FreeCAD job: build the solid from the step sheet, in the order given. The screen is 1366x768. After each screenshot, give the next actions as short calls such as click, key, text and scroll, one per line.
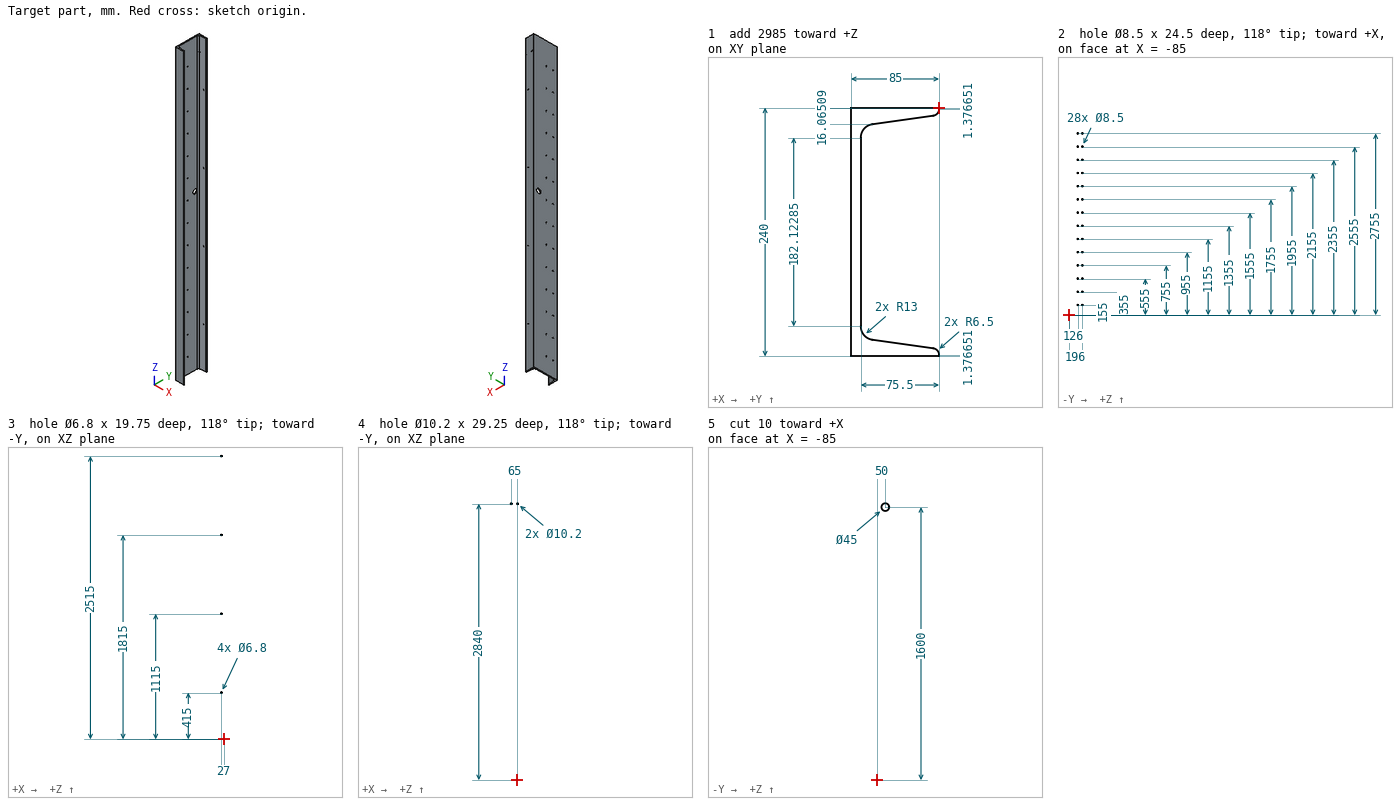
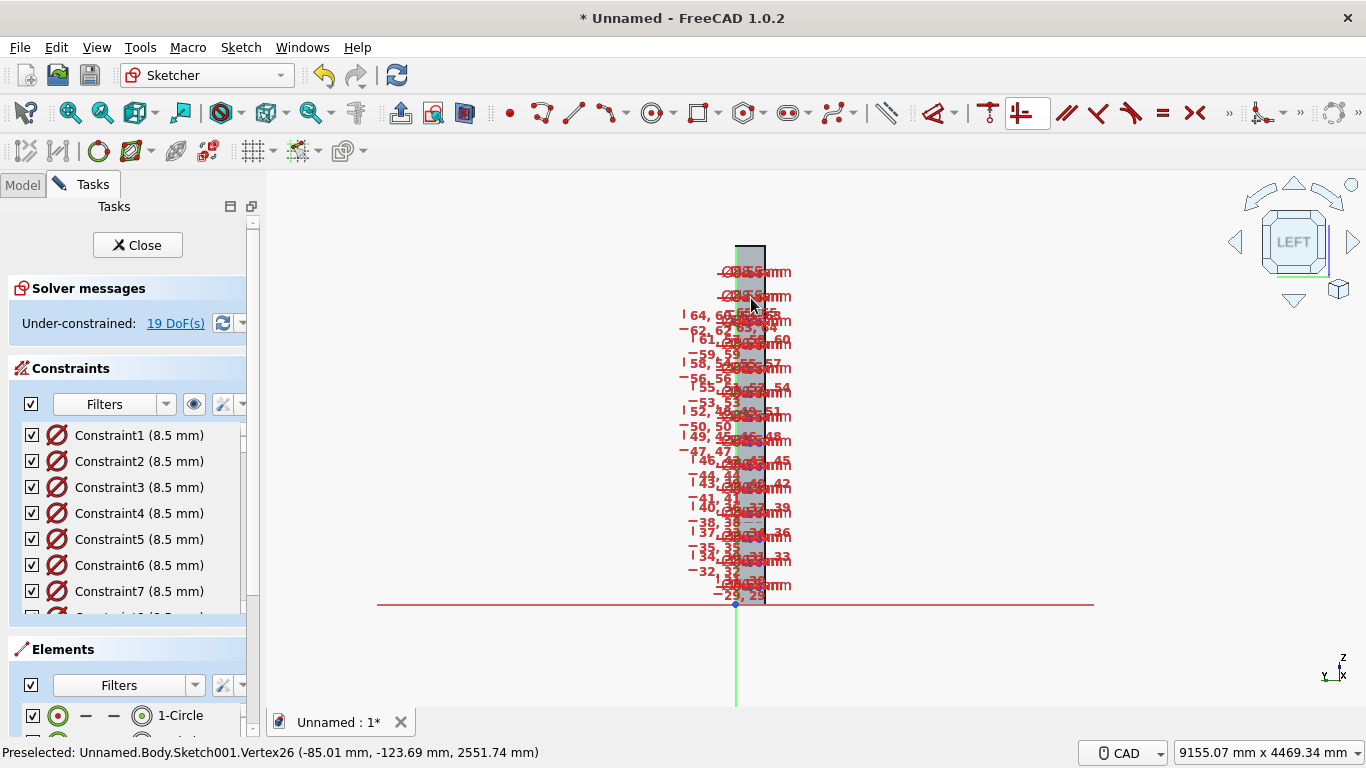
scroll(751, 298, up, 2)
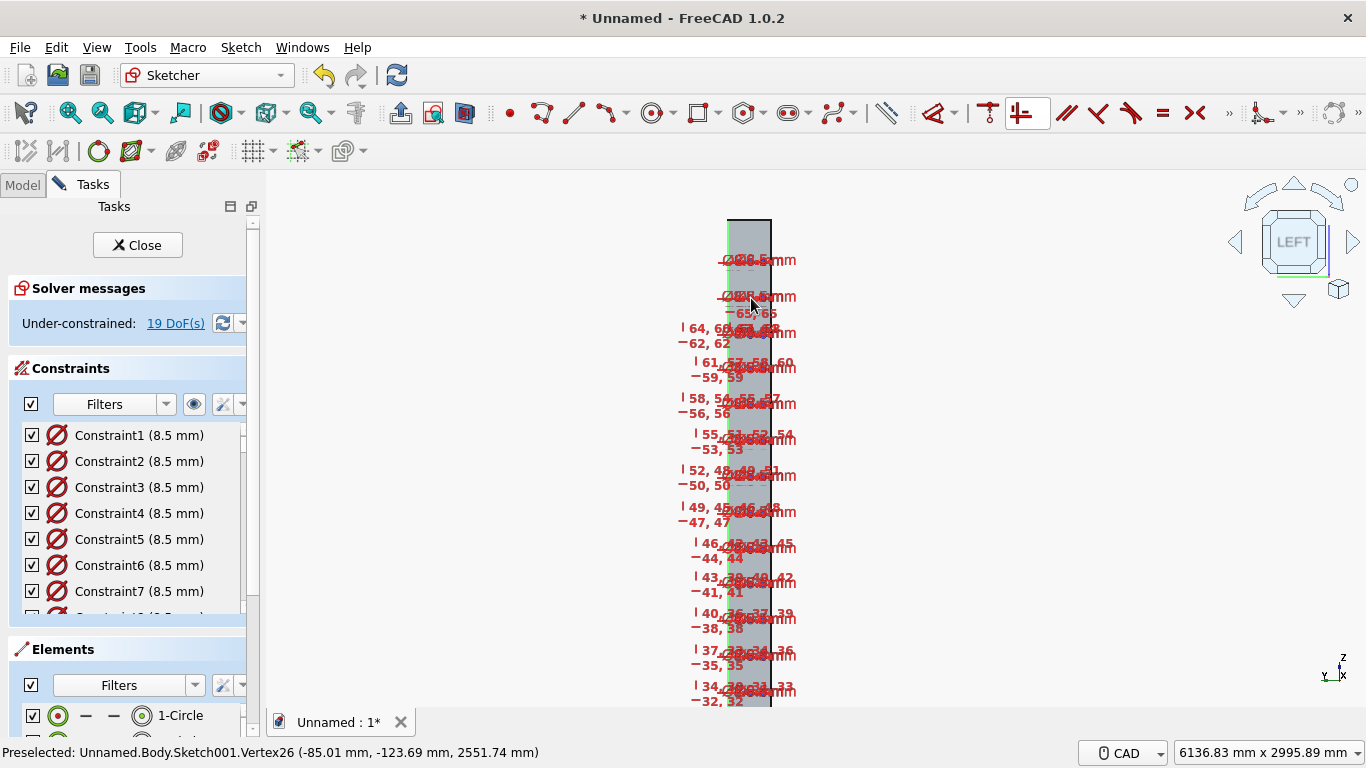
click(750, 299)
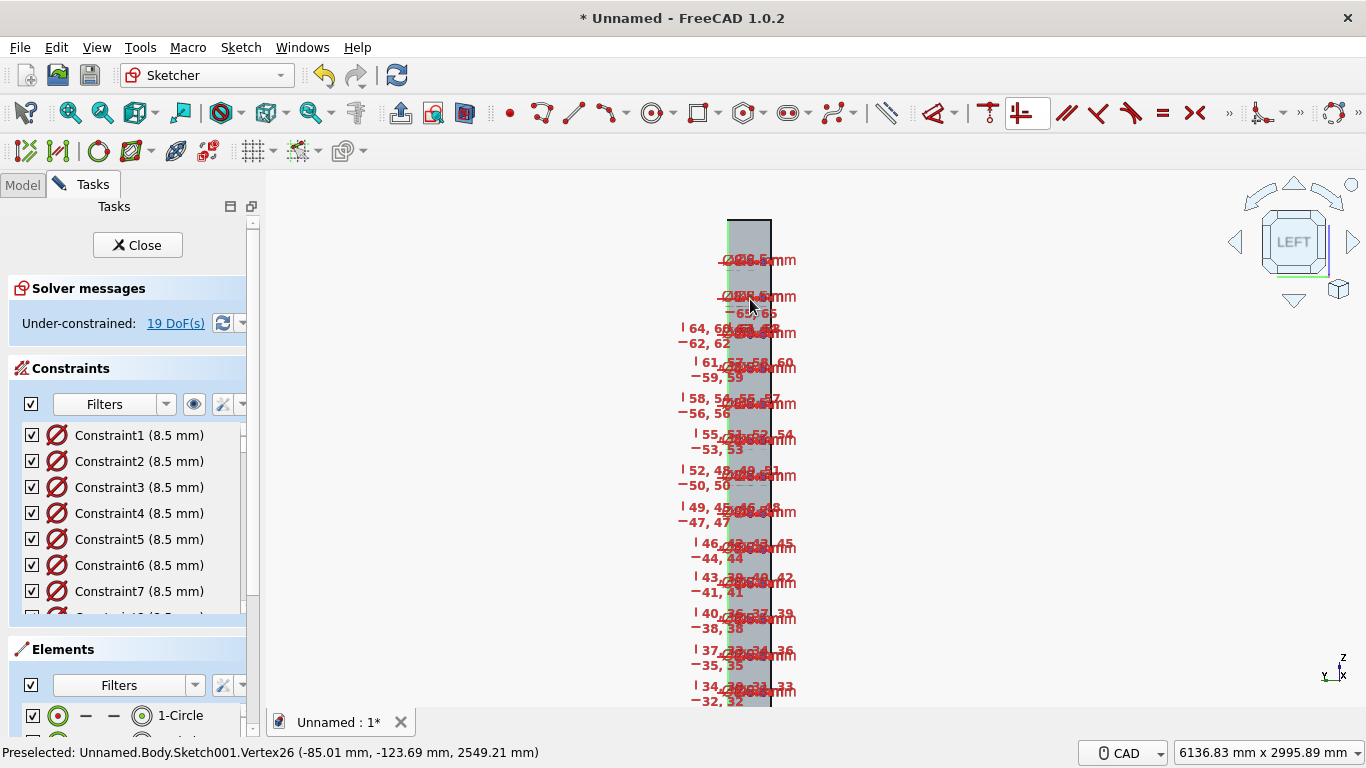
click(751, 263)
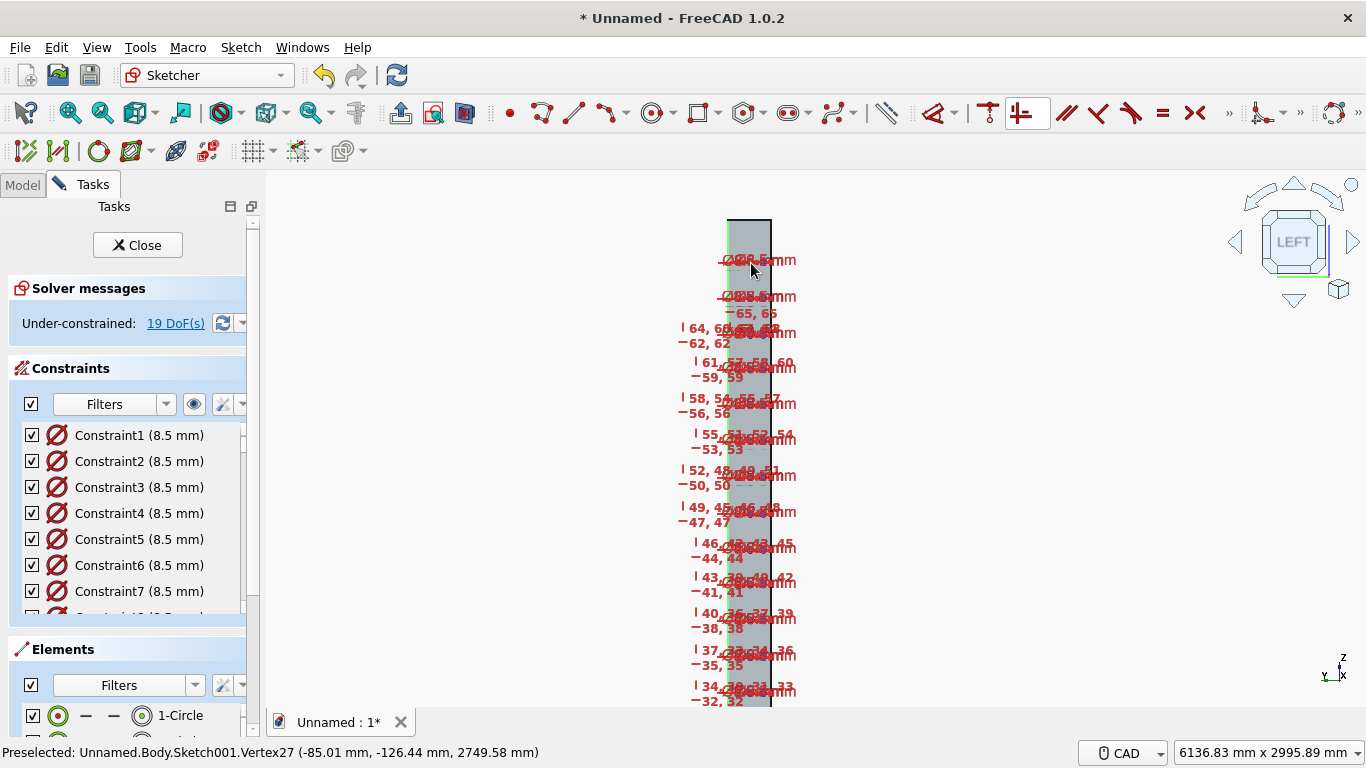
key(v)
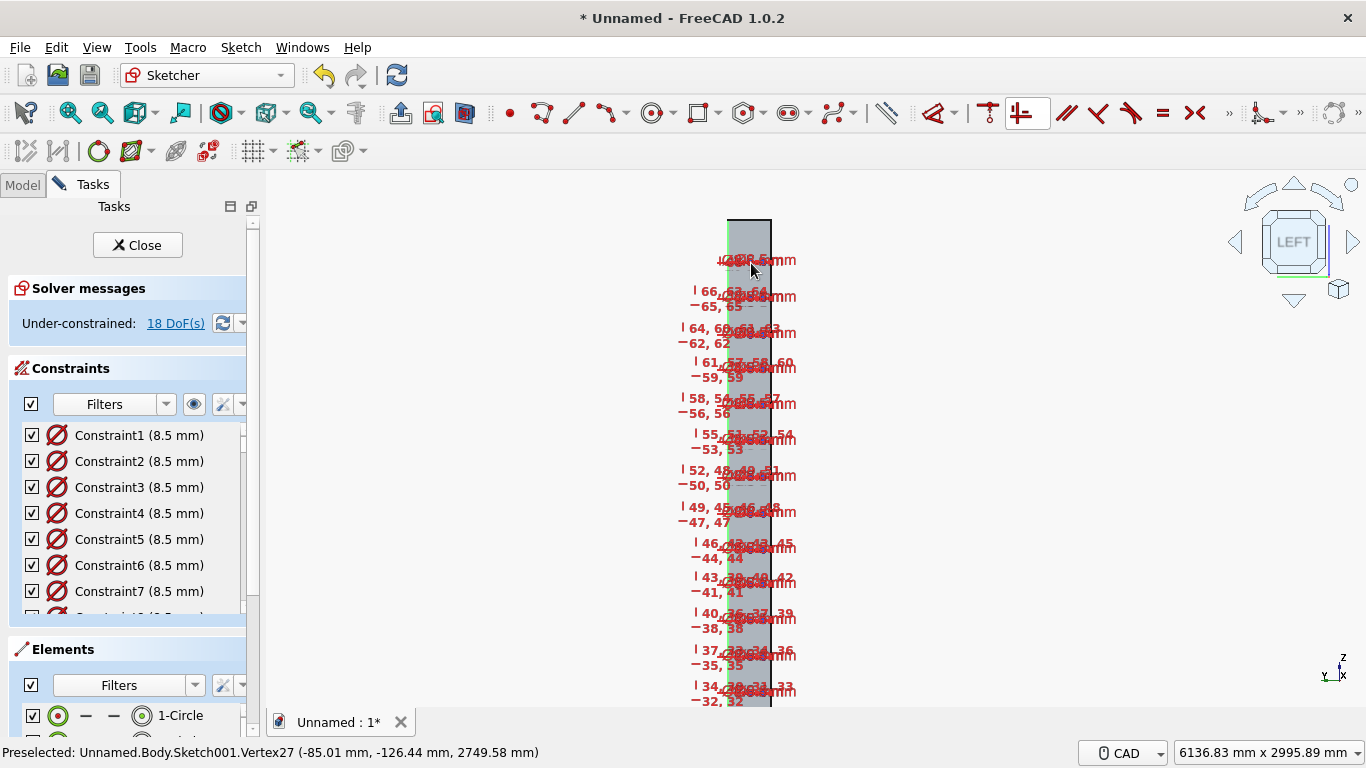
click(763, 299)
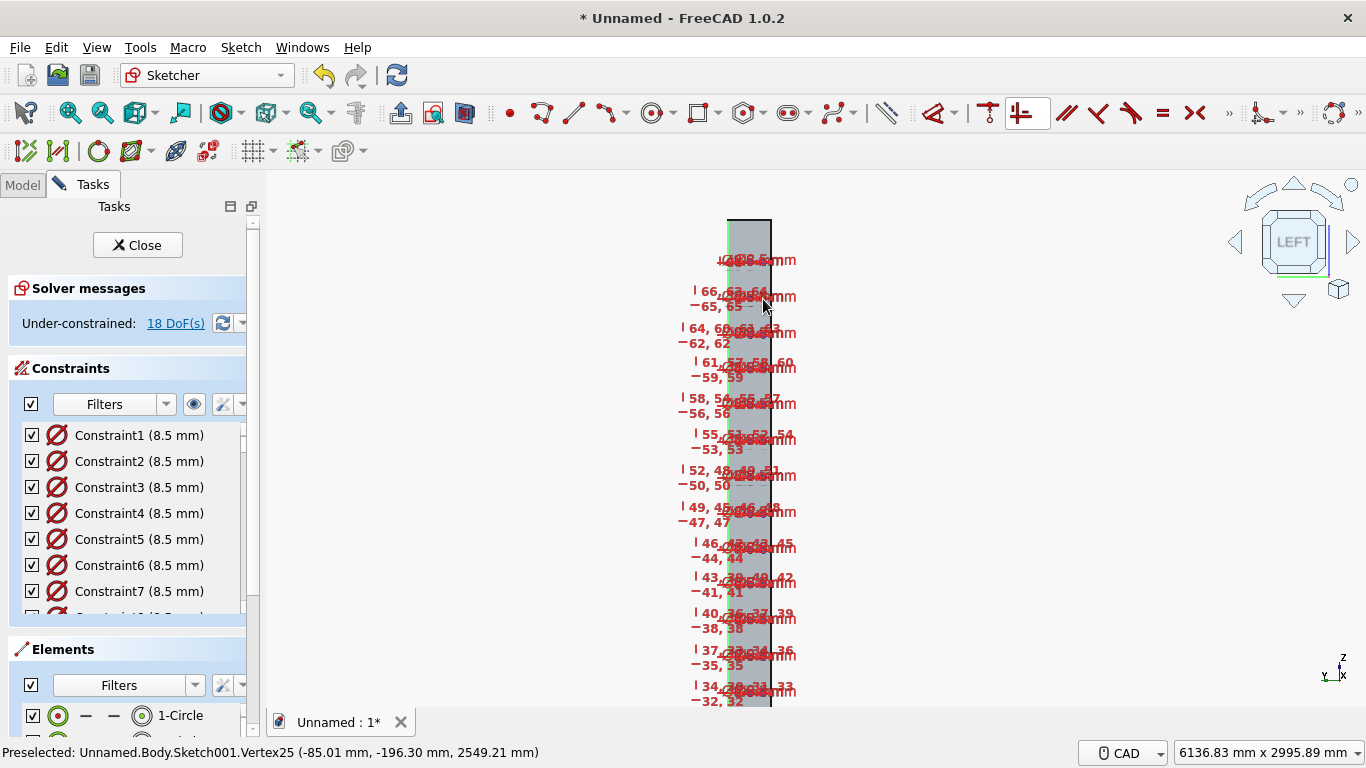
click(763, 262)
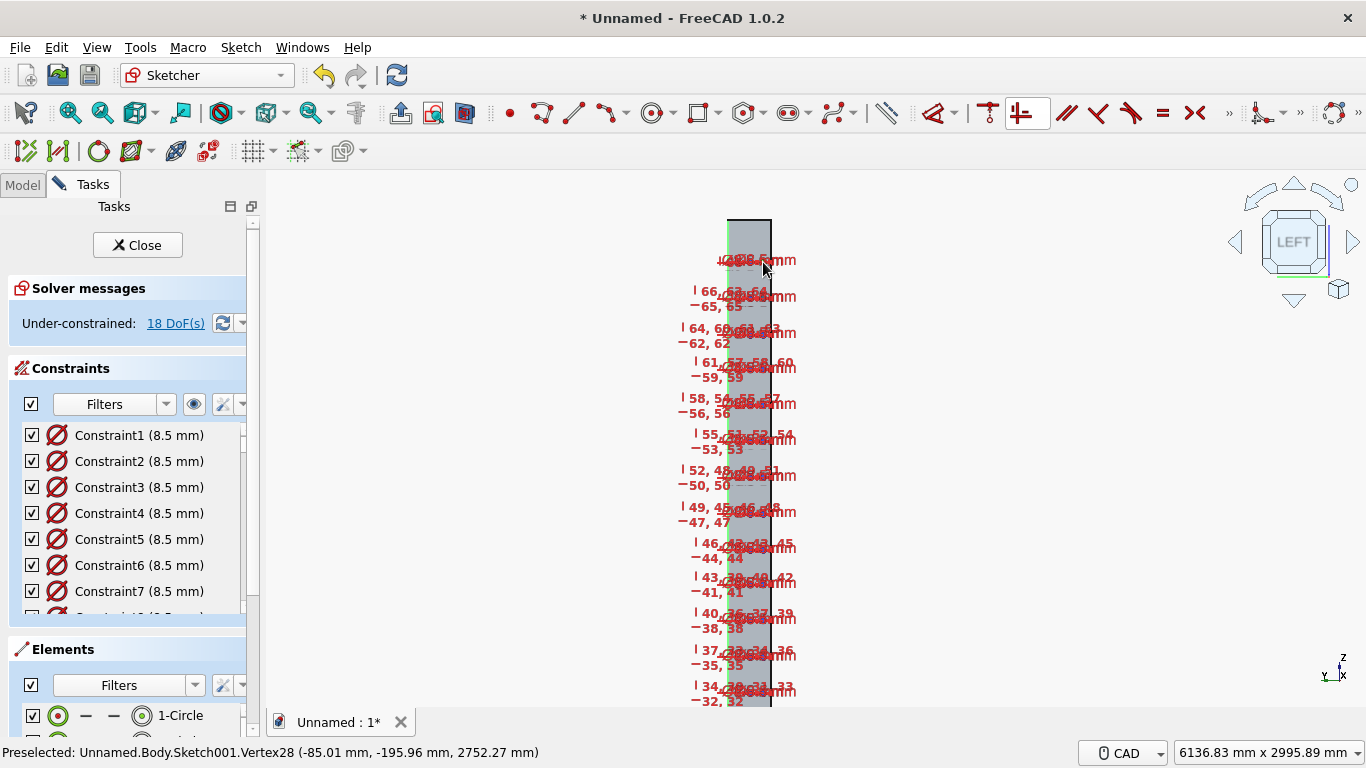
click(1044, 114)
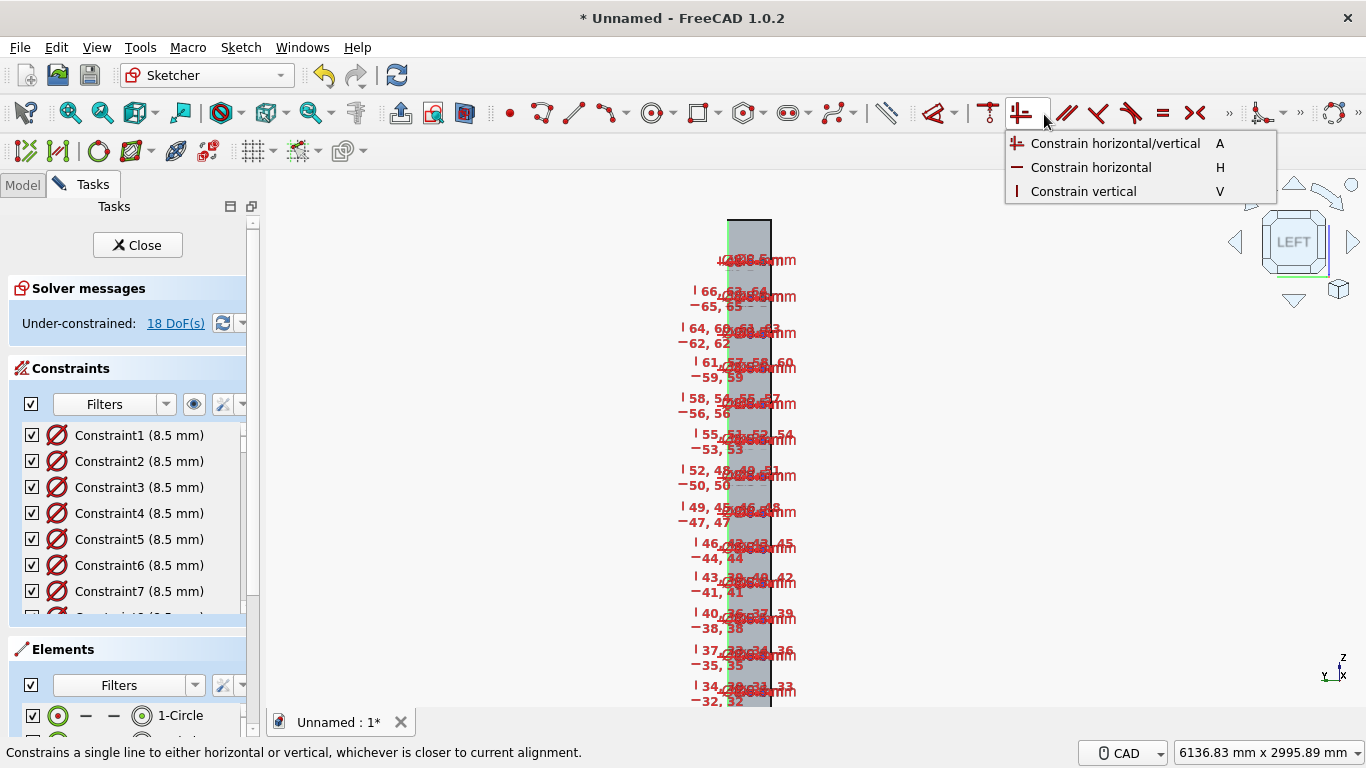
click(1141, 191)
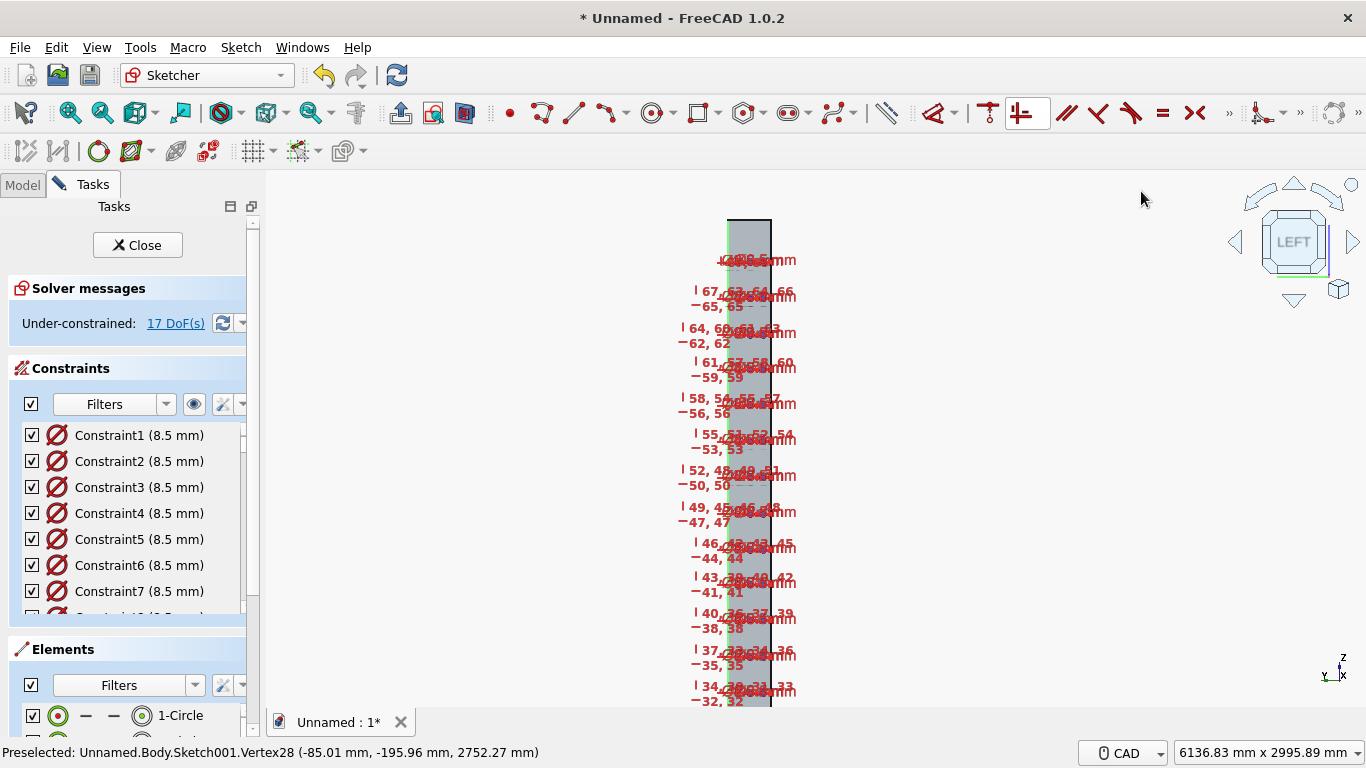
scroll(750, 263, up, 4)